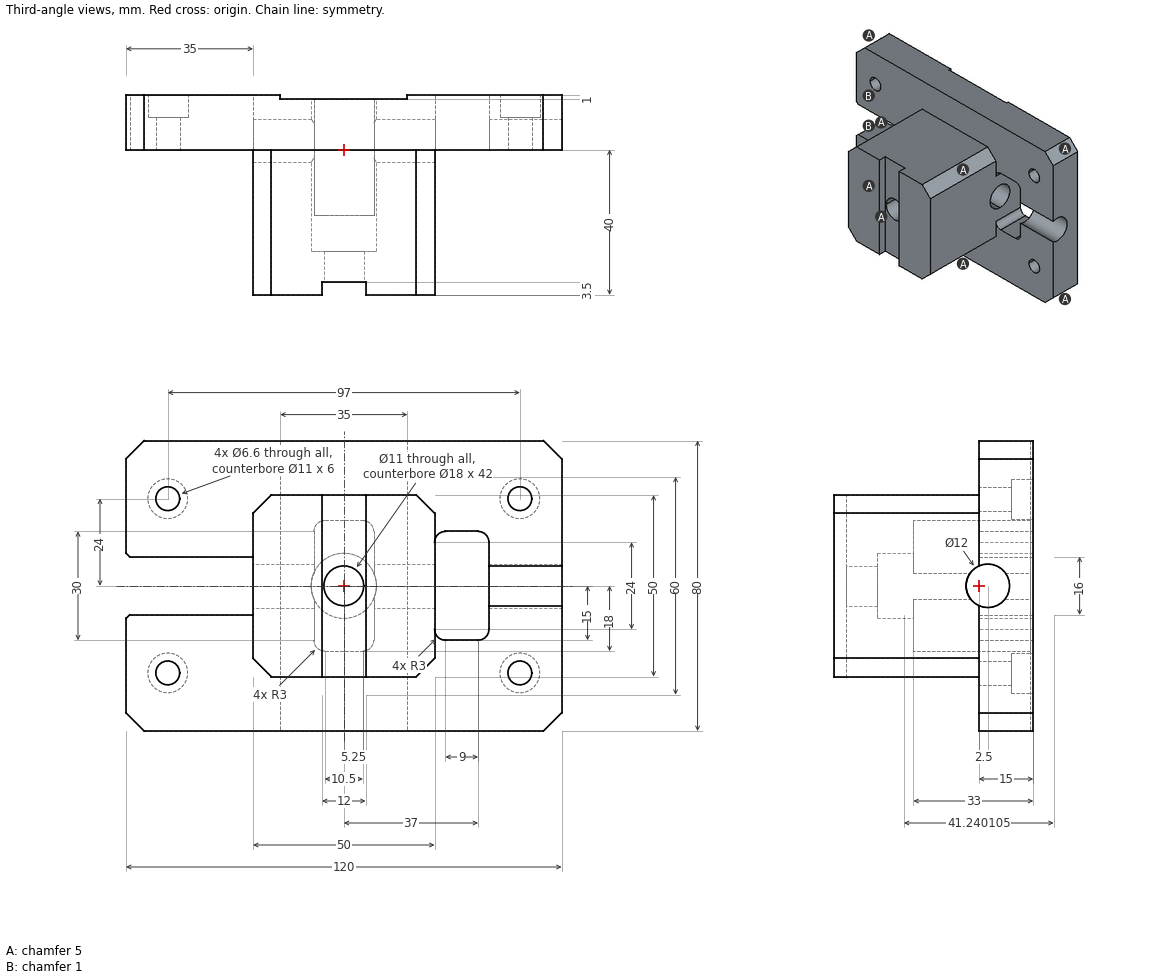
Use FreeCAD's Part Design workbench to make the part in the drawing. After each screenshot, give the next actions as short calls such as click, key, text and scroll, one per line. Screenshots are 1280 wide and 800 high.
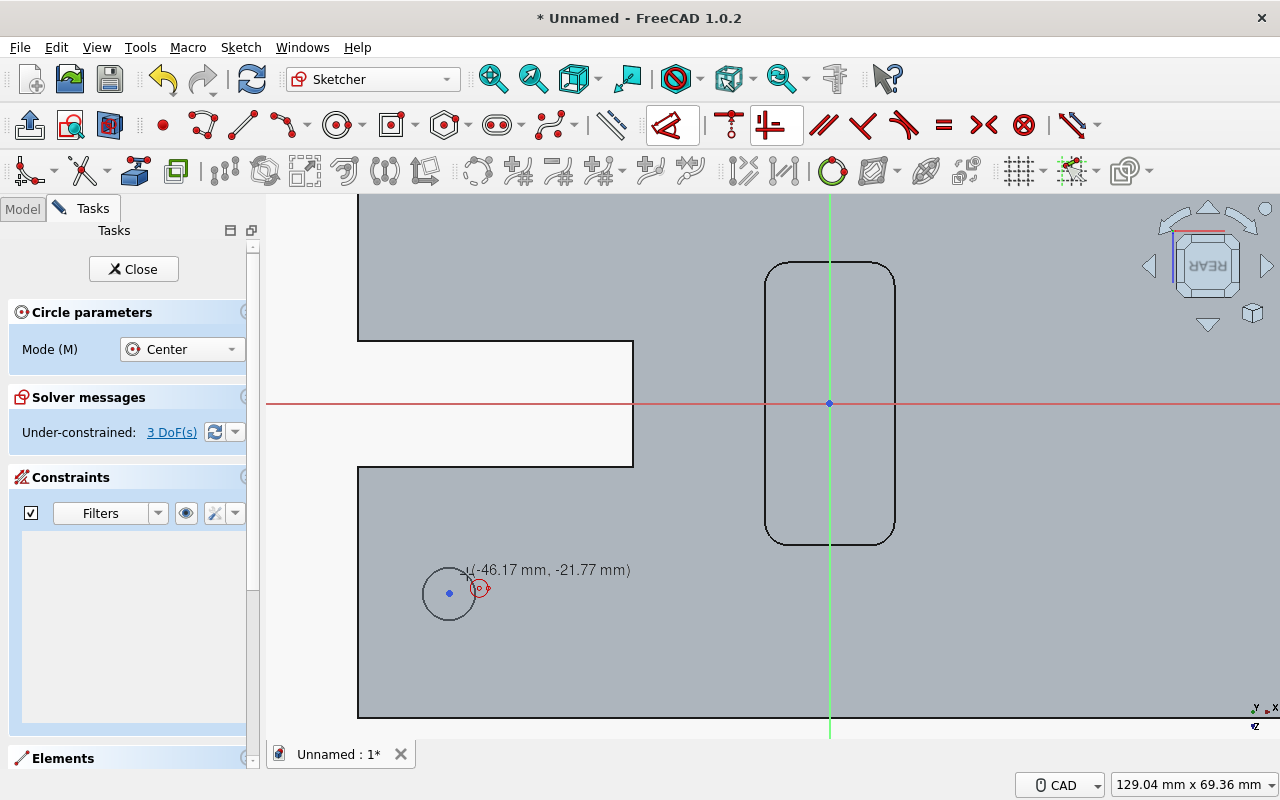
scroll(450, 594, down, 2)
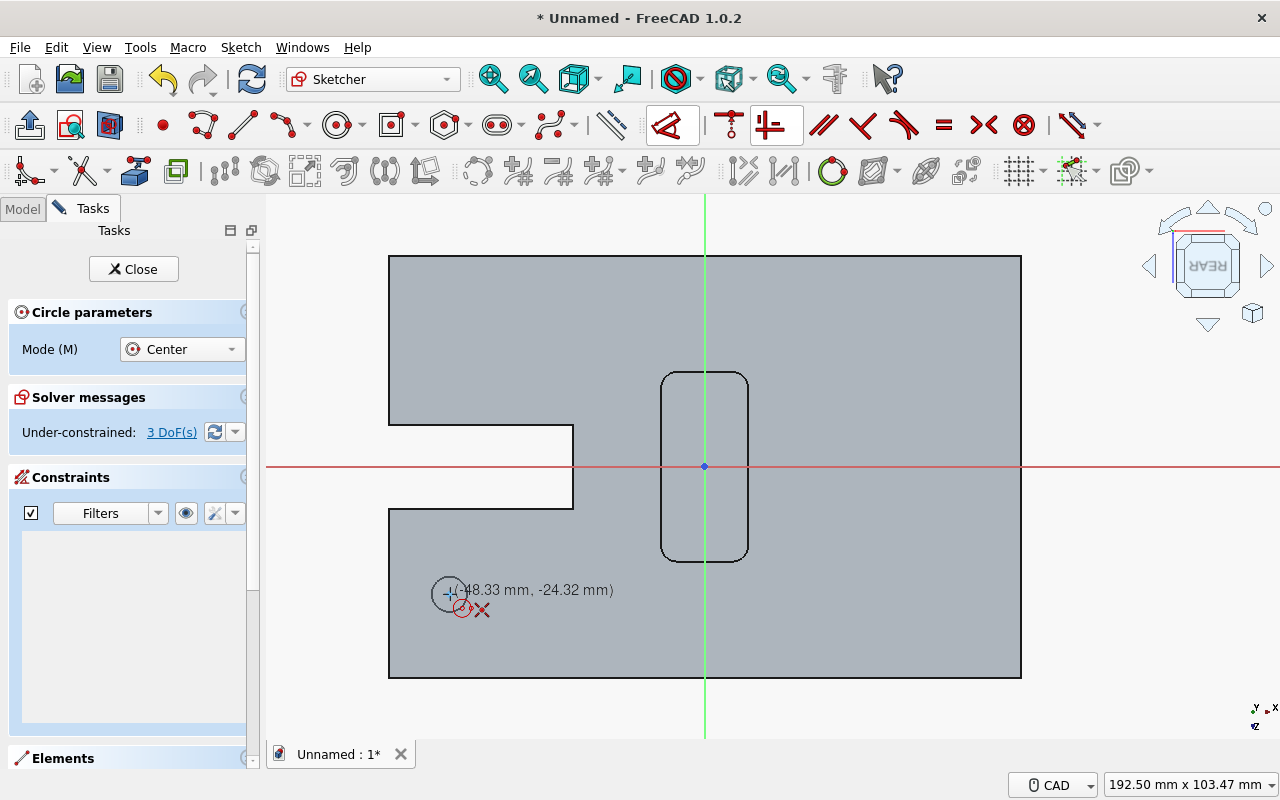
scroll(960, 593, up, 2)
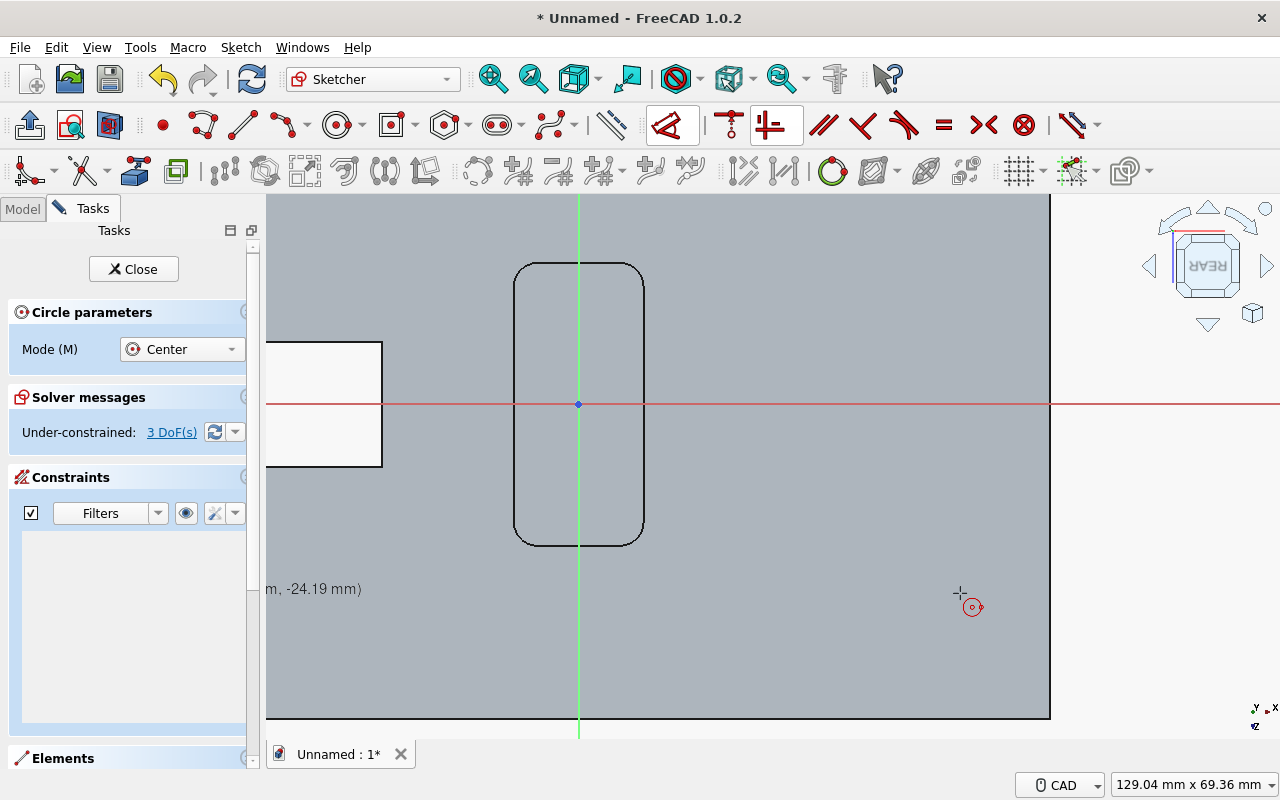
click(960, 593)
click(978, 575)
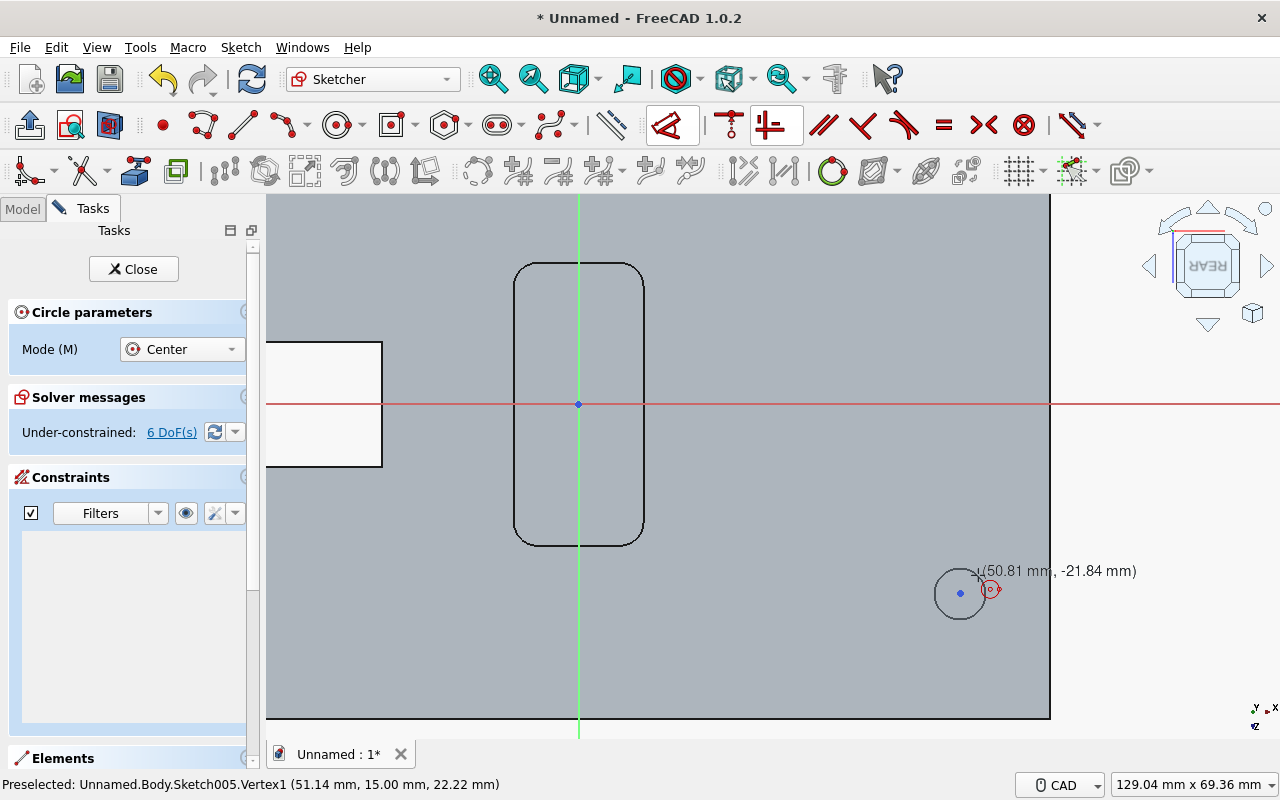
scroll(960, 593, down, 2)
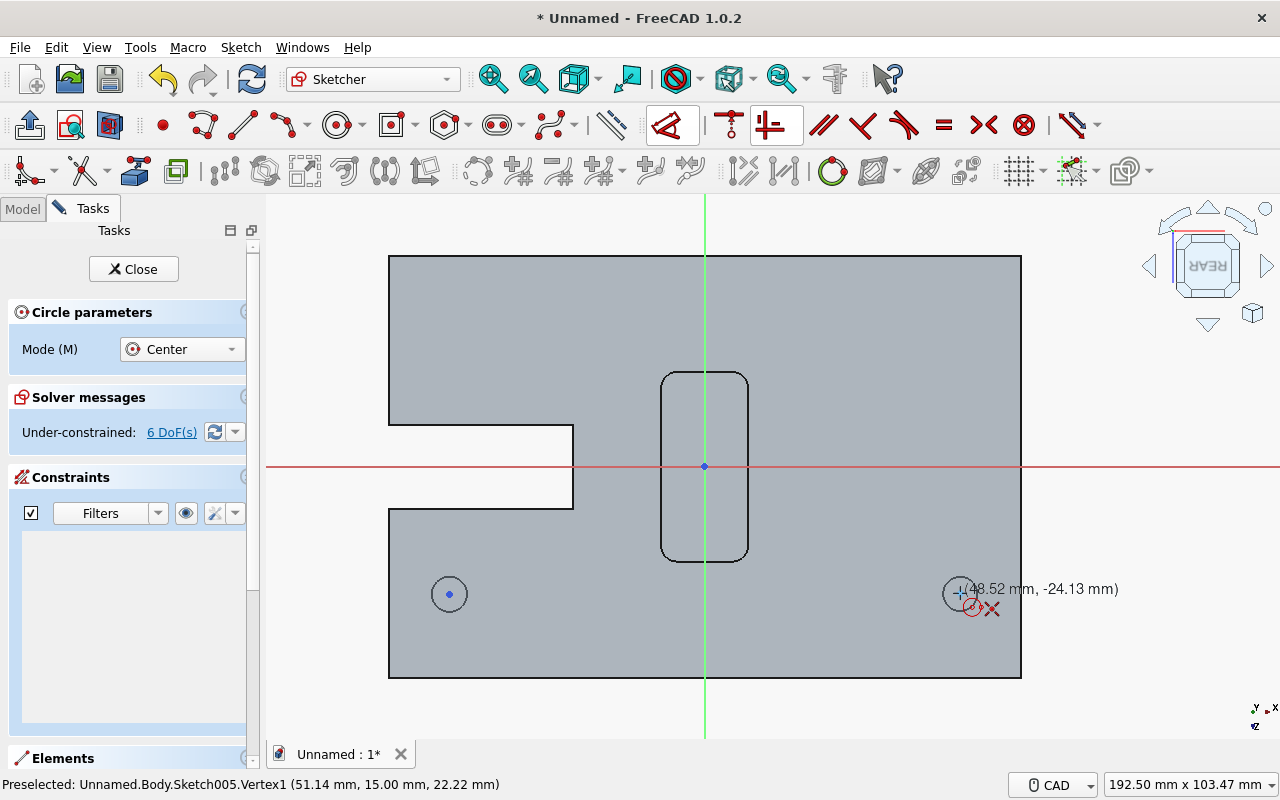
scroll(960, 340, up, 2)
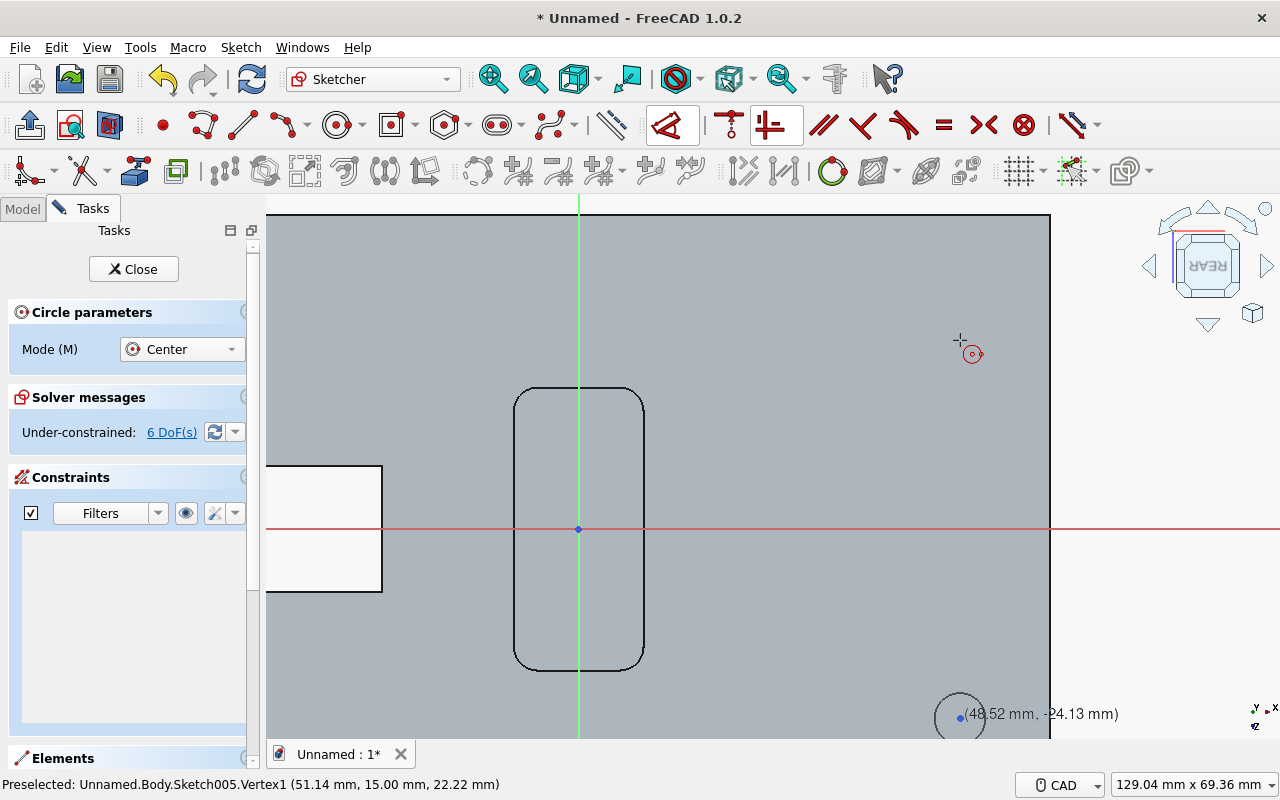
click(960, 340)
click(978, 322)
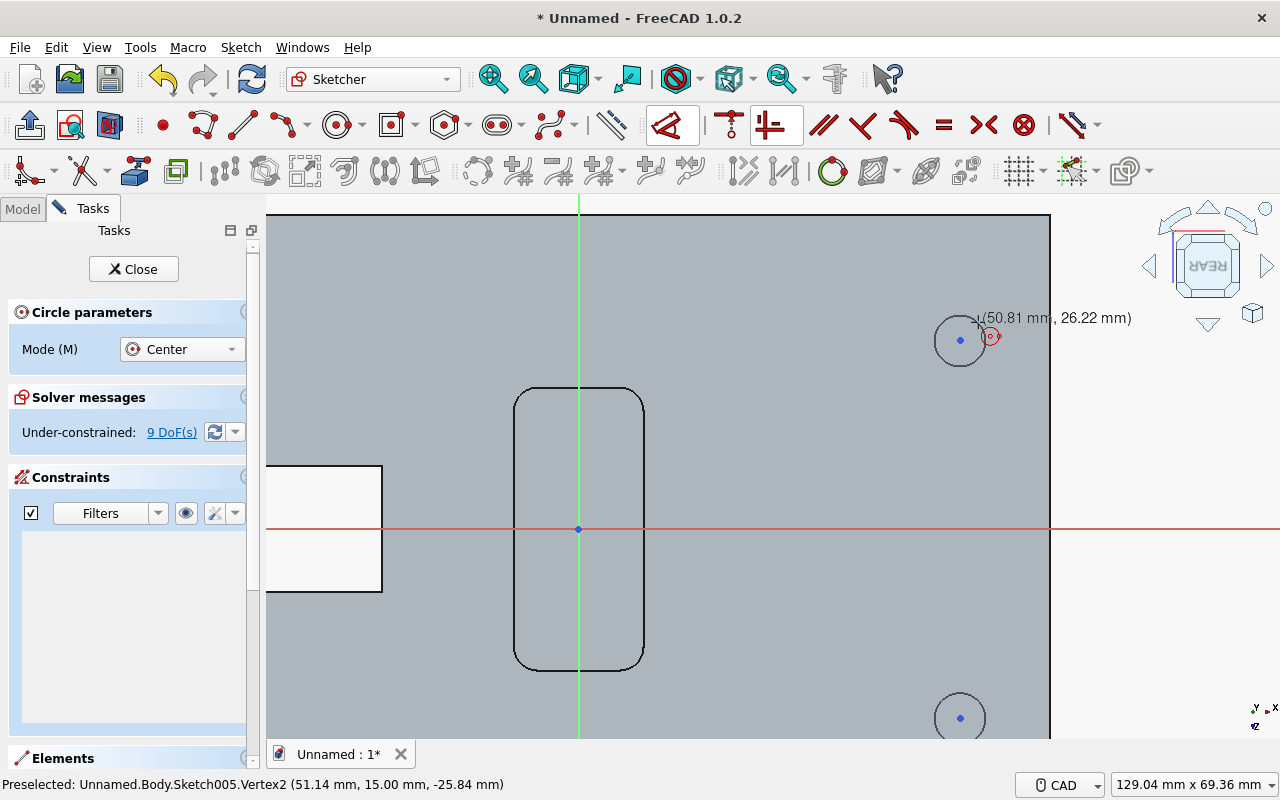
scroll(960, 339, down, 2)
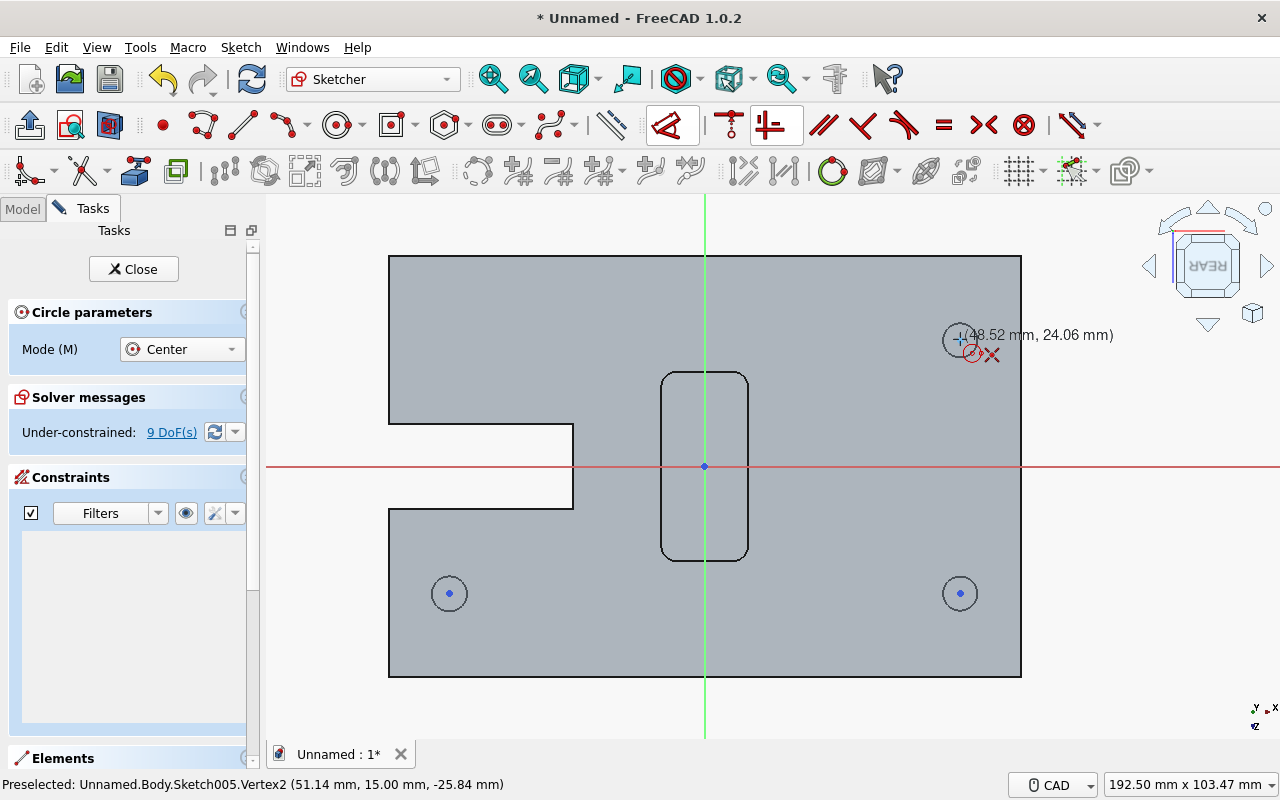
scroll(449, 340, up, 2)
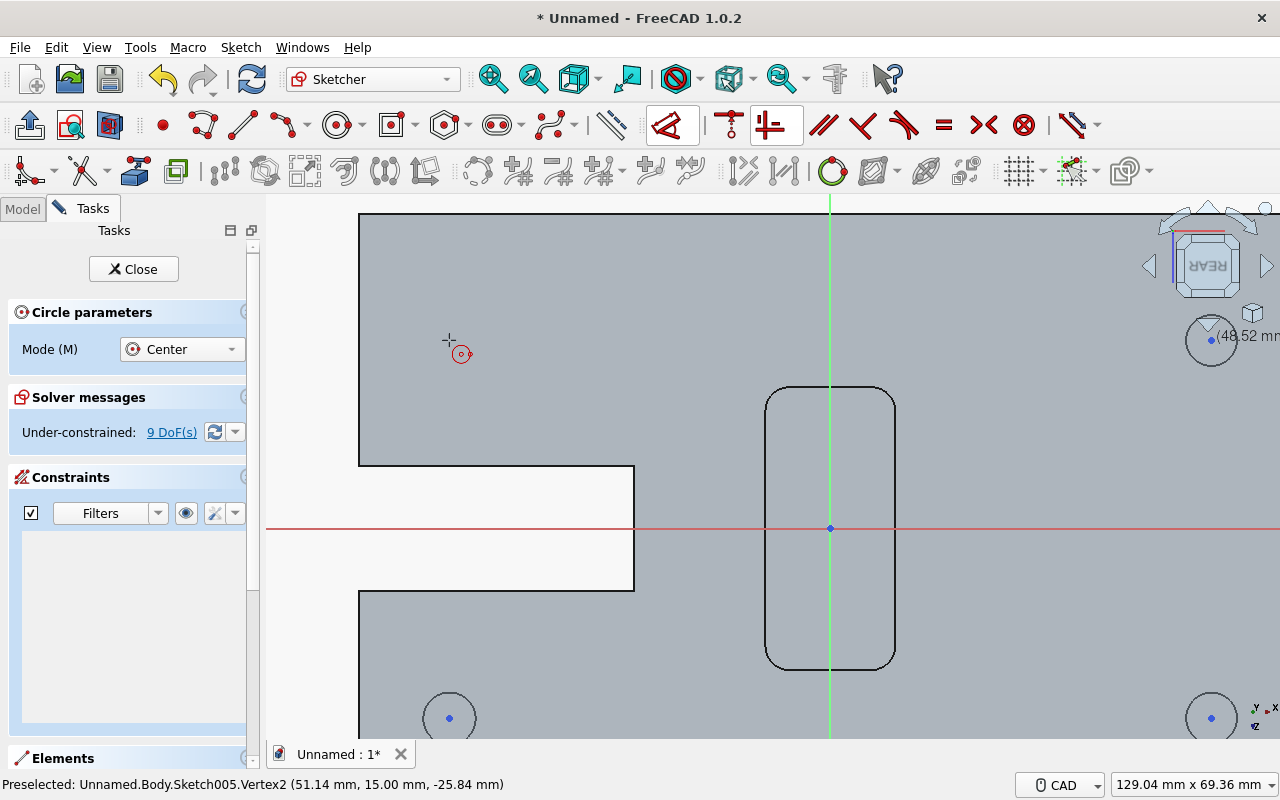
click(449, 340)
click(468, 322)
key(Escape)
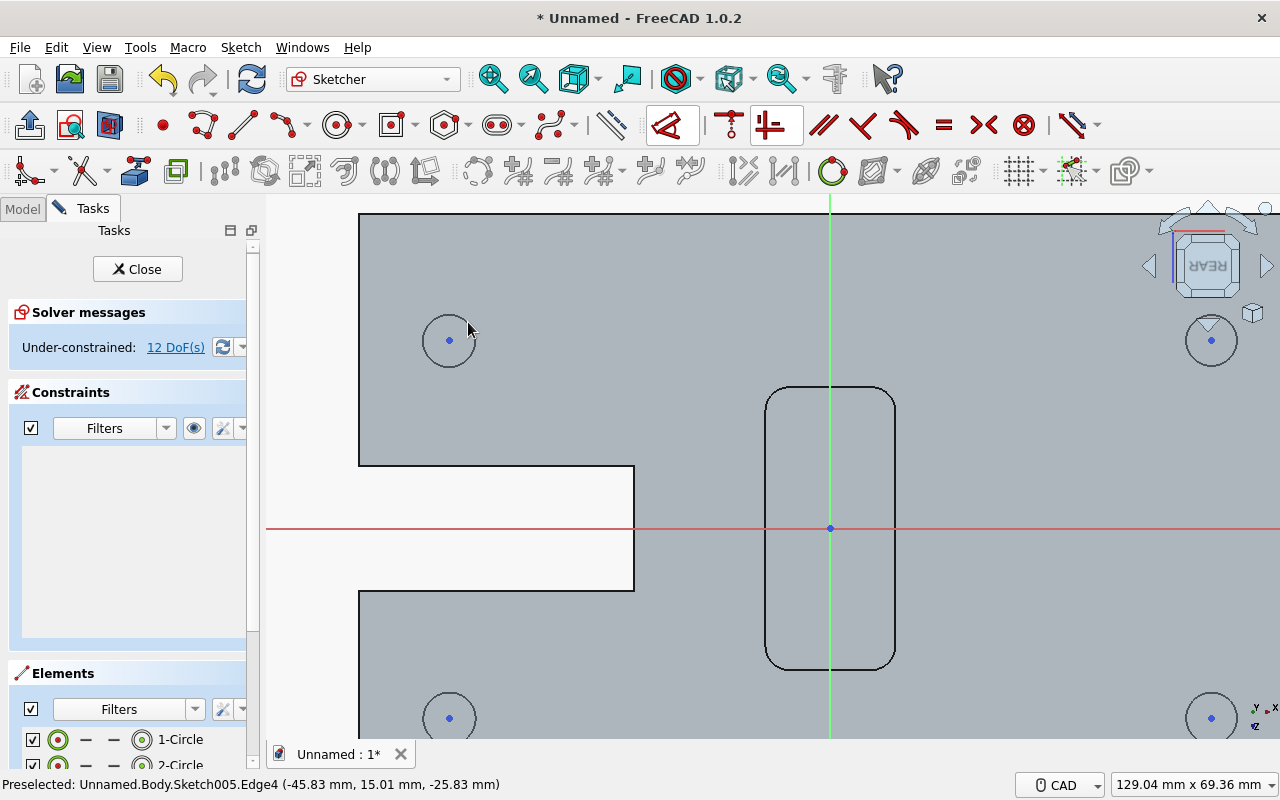
click(468, 700)